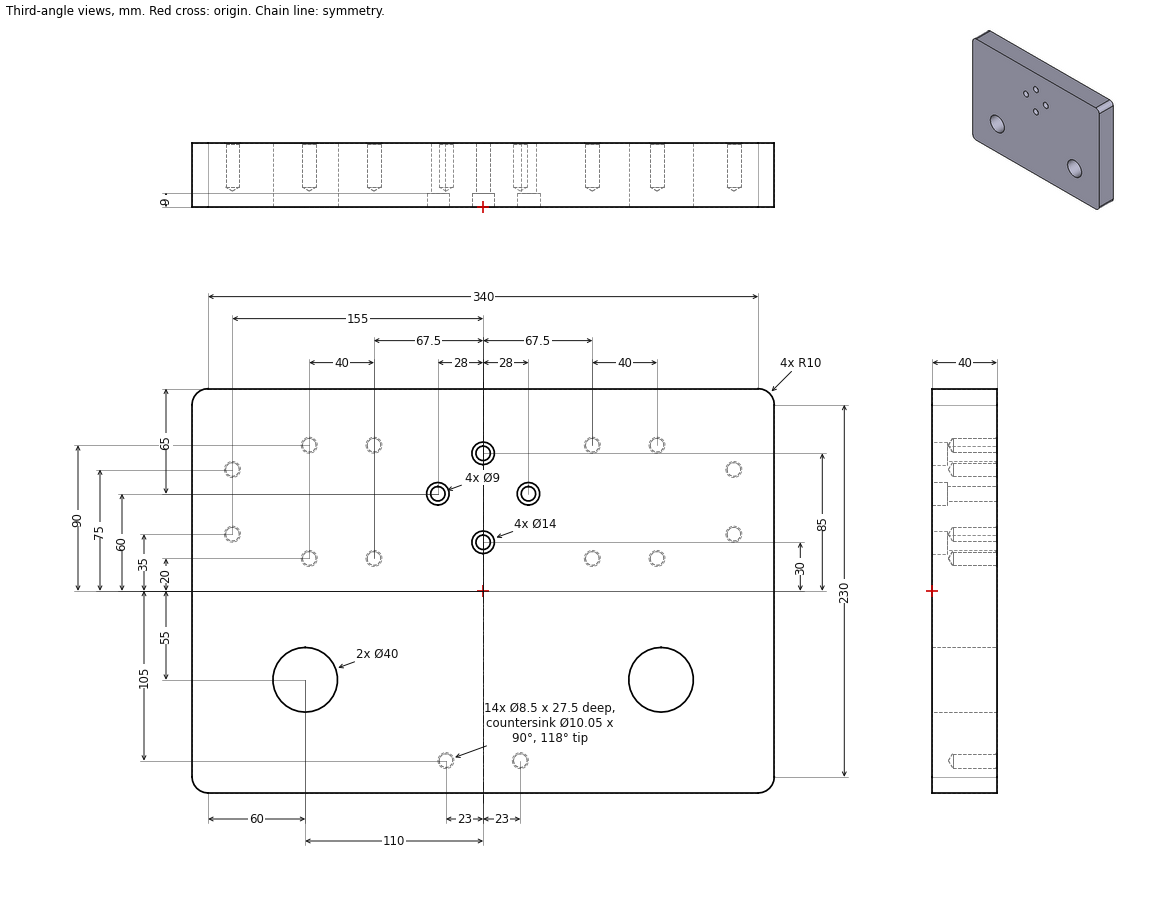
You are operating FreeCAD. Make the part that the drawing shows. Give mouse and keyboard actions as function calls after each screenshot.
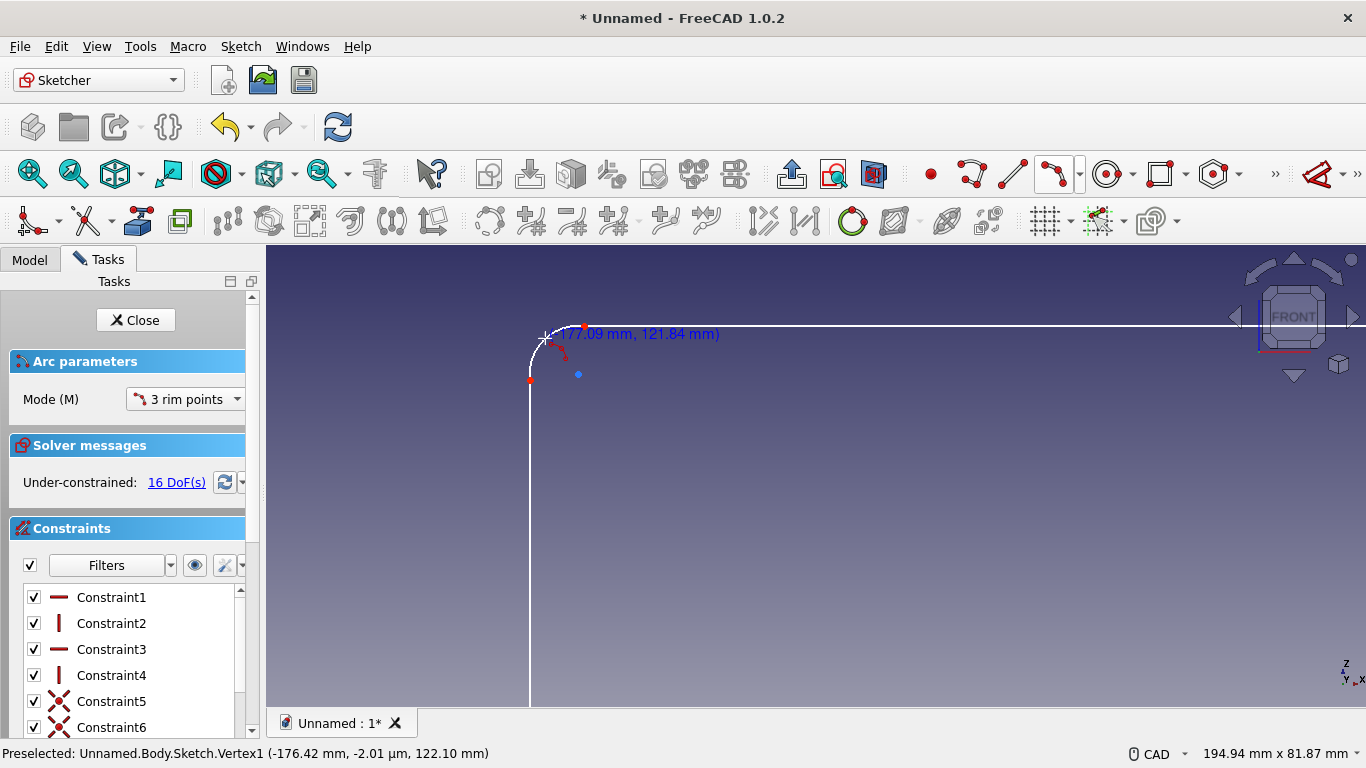
click(1106, 174)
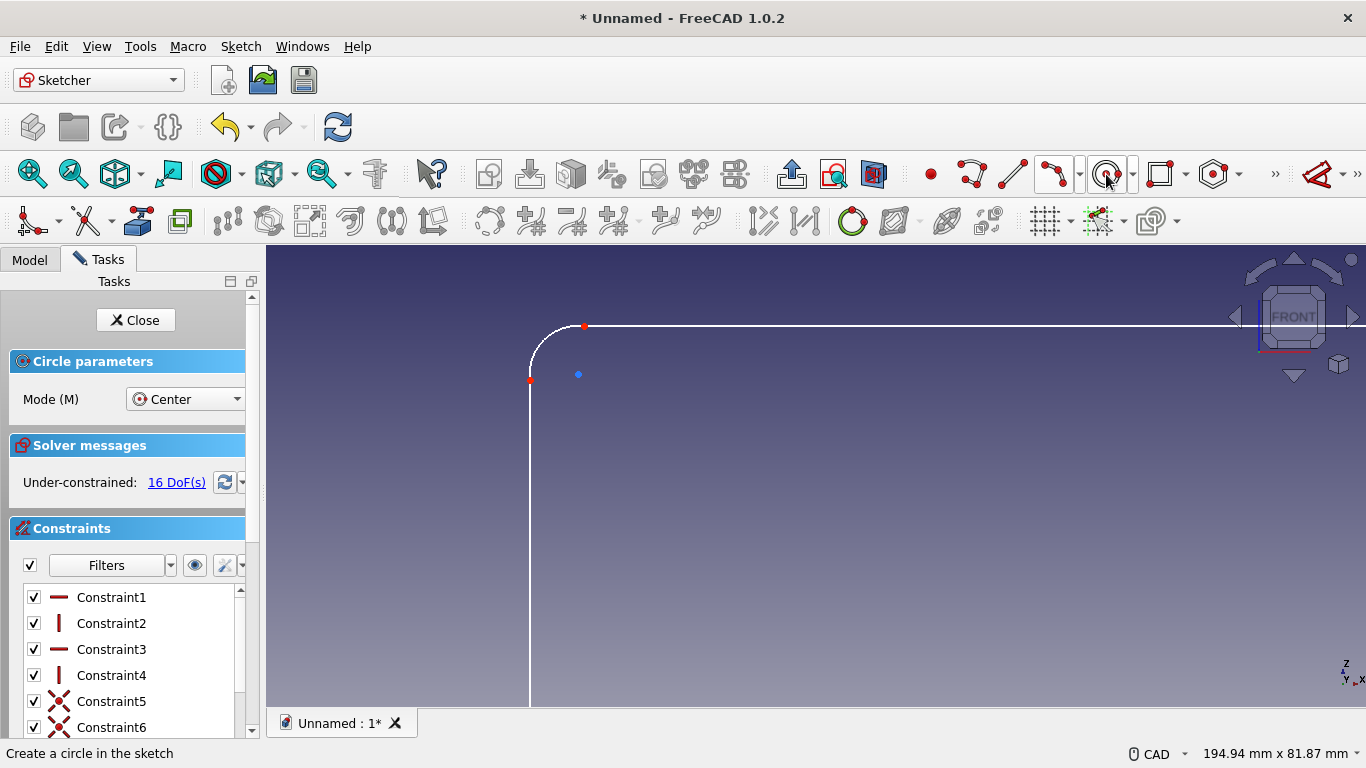
scroll(546, 337, down, 8)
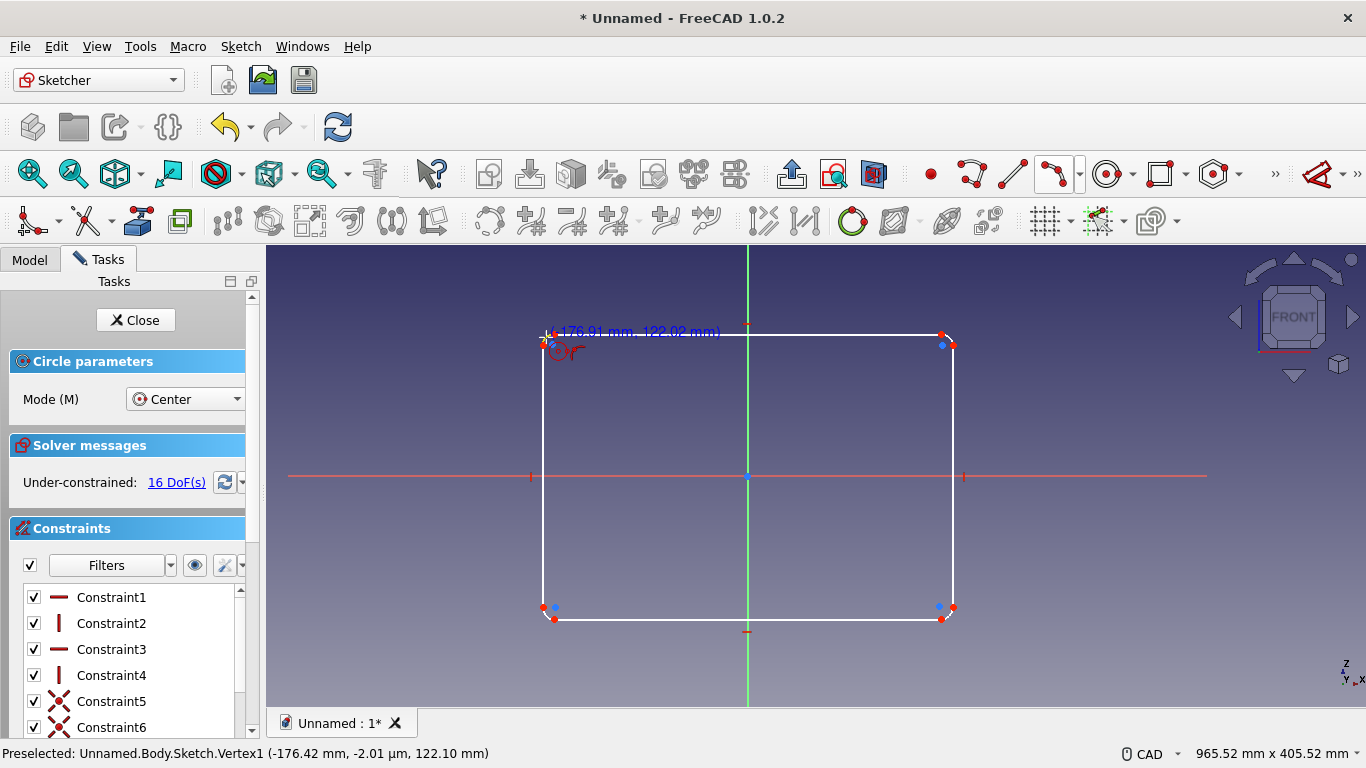
scroll(716, 408, up, 8)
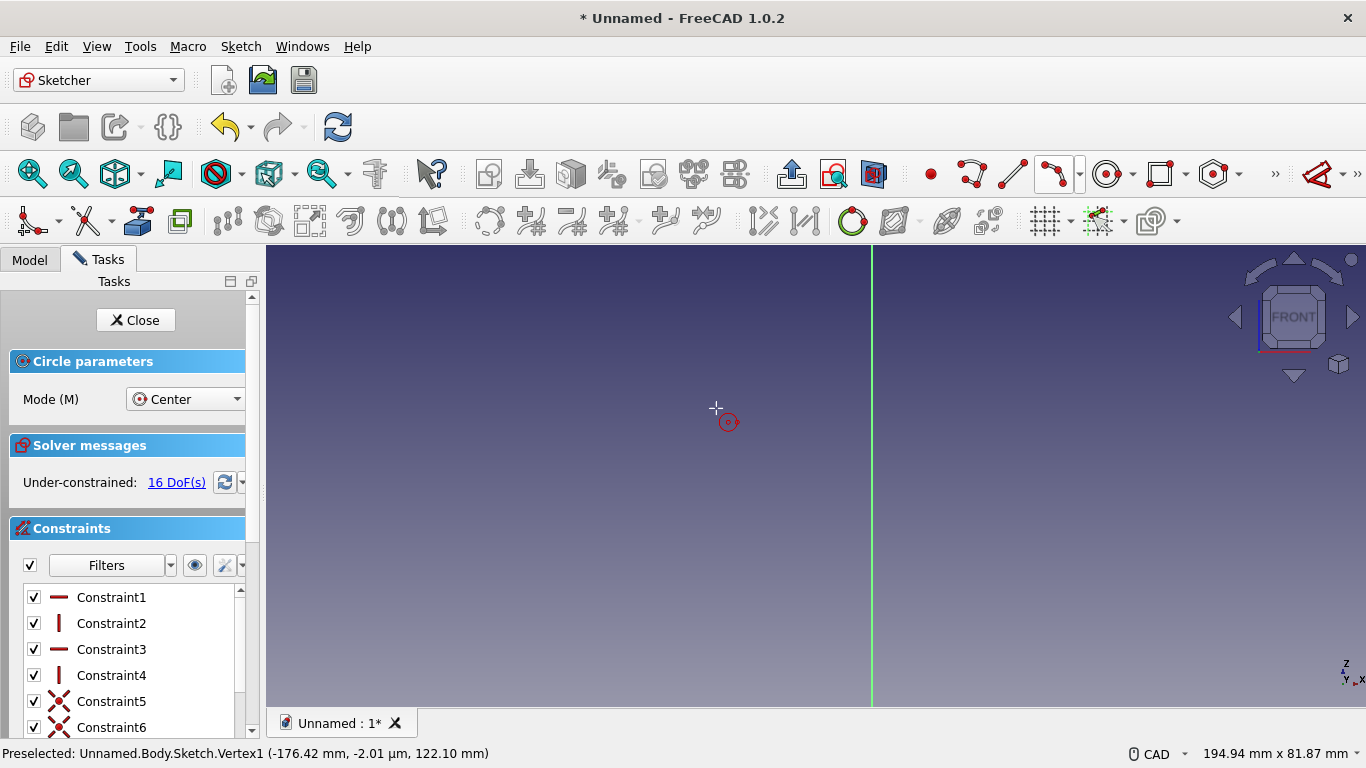
scroll(716, 408, down, 8)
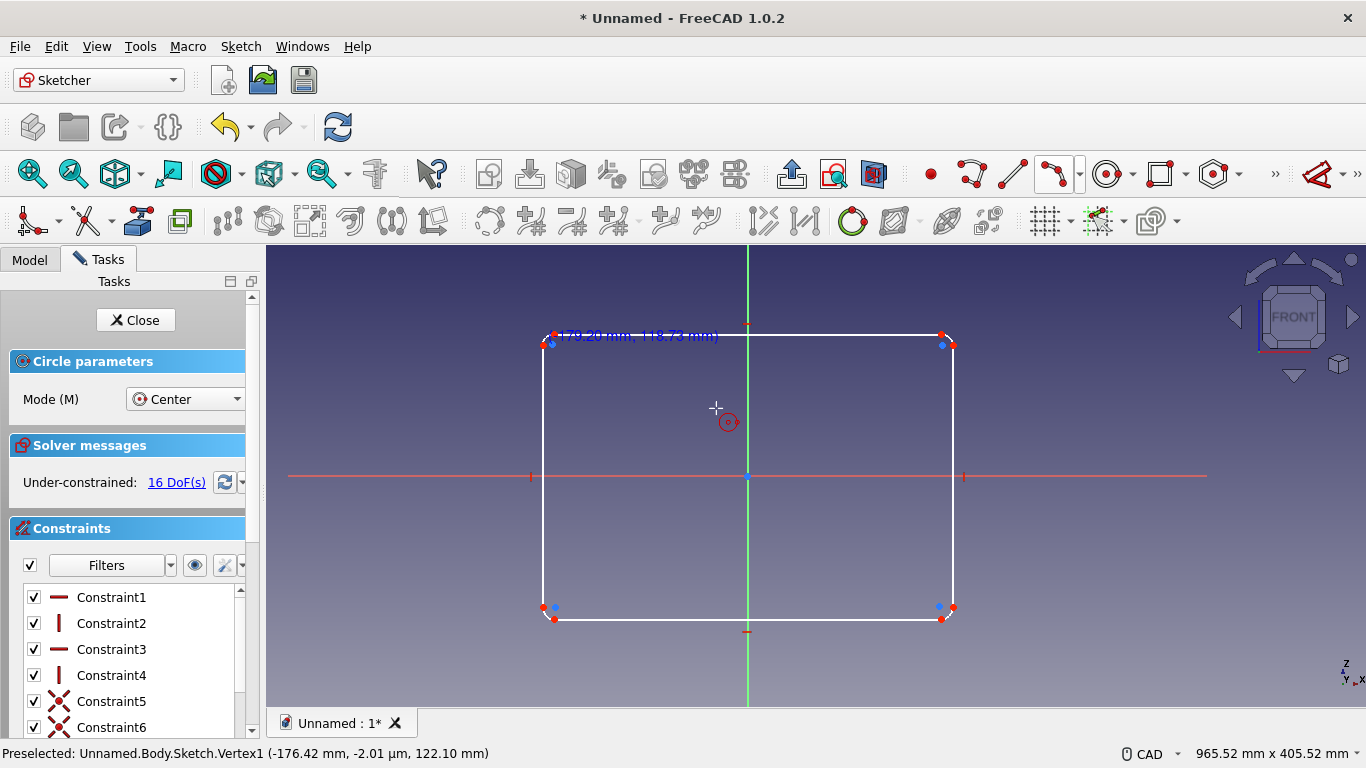
click(716, 408)
move(719, 404)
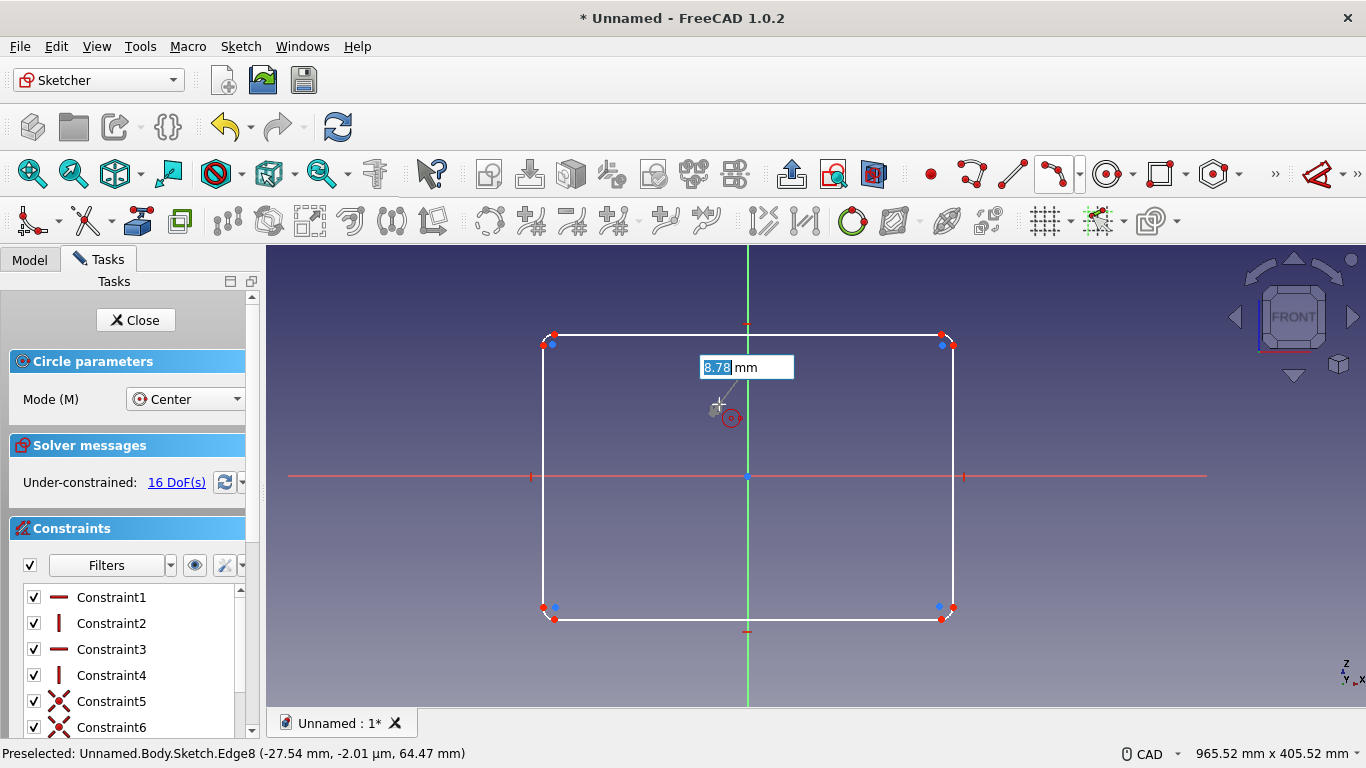
text(9)
key(Return)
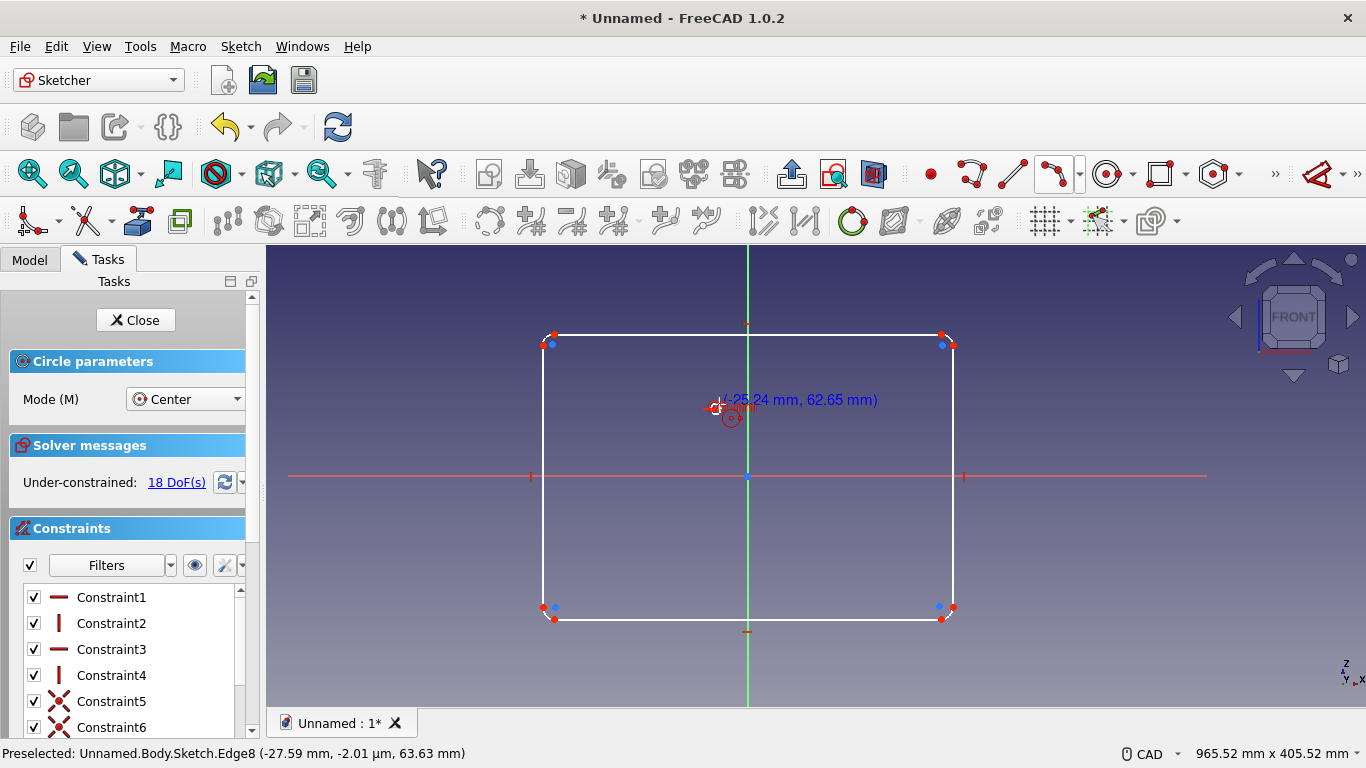
scroll(748, 380, up, 8)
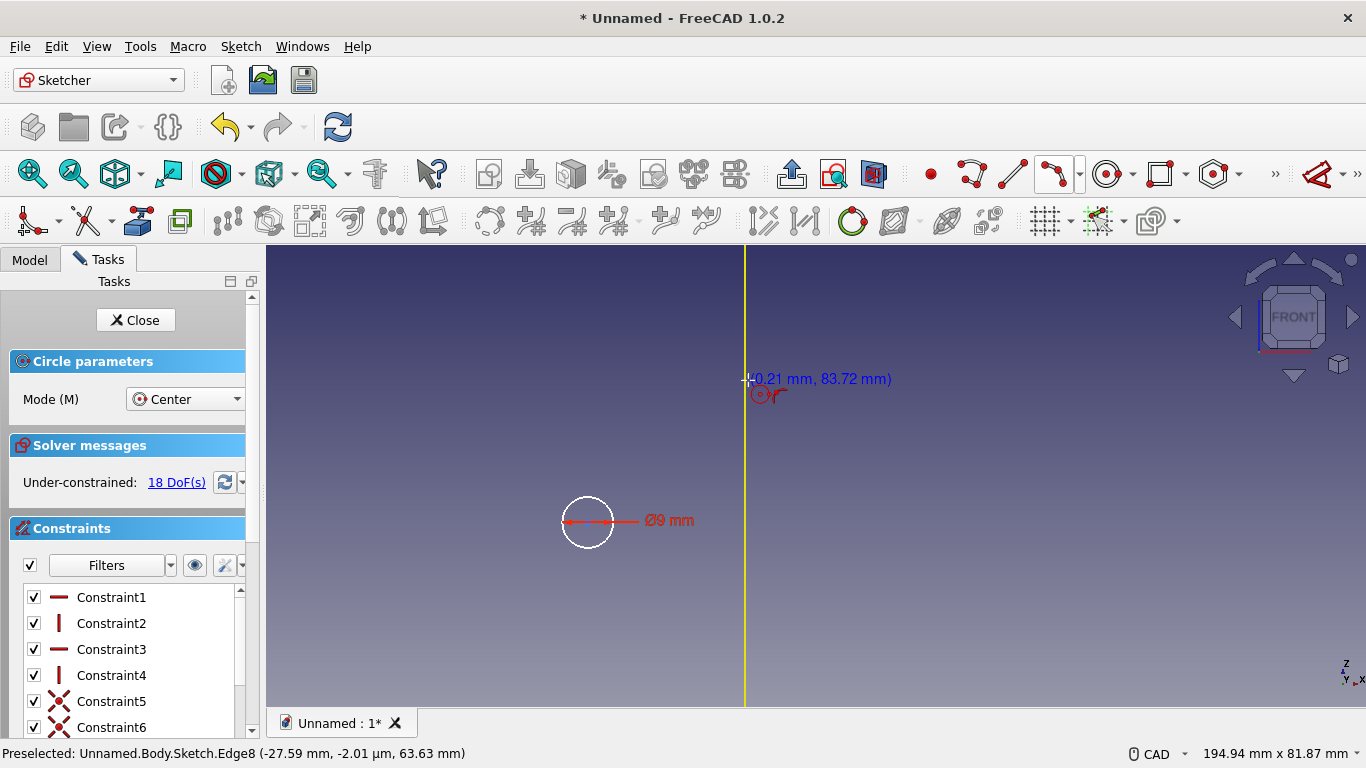
scroll(748, 380, down, 8)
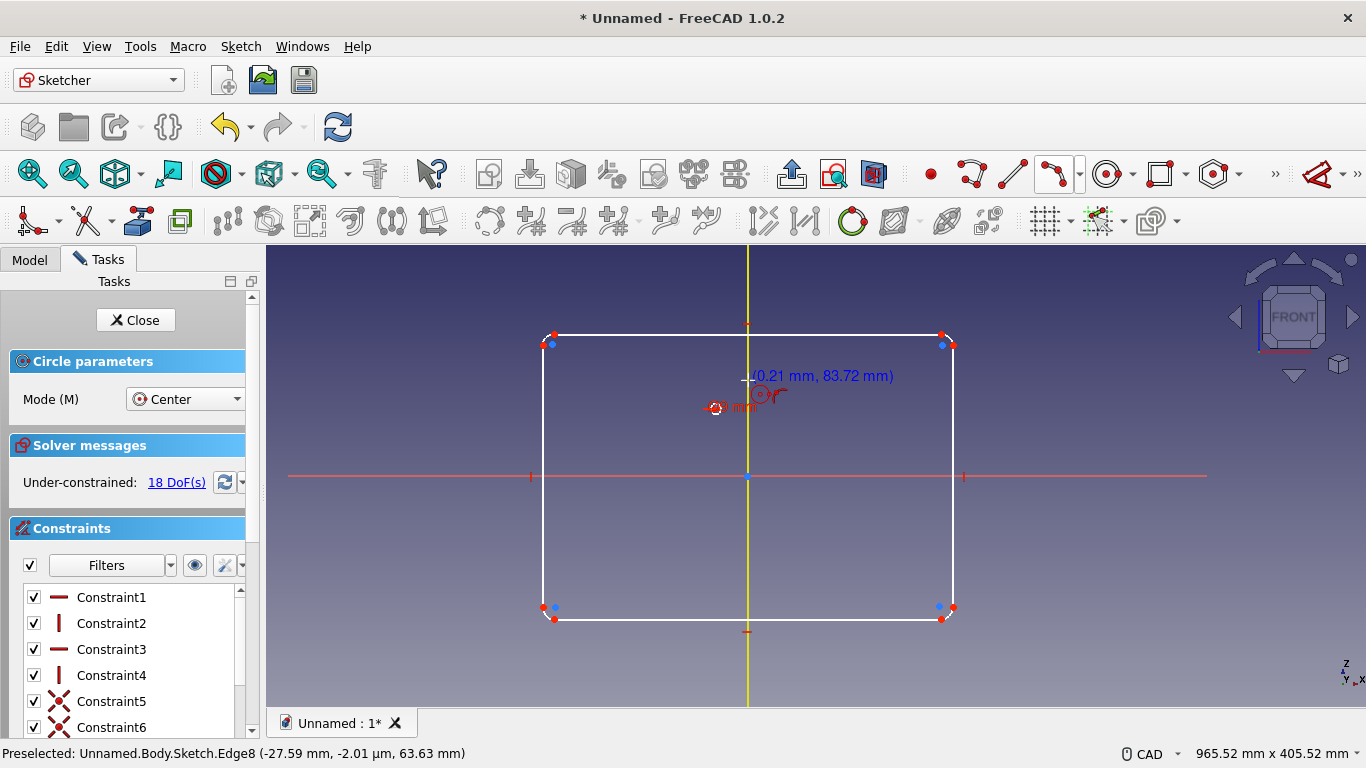
click(748, 380)